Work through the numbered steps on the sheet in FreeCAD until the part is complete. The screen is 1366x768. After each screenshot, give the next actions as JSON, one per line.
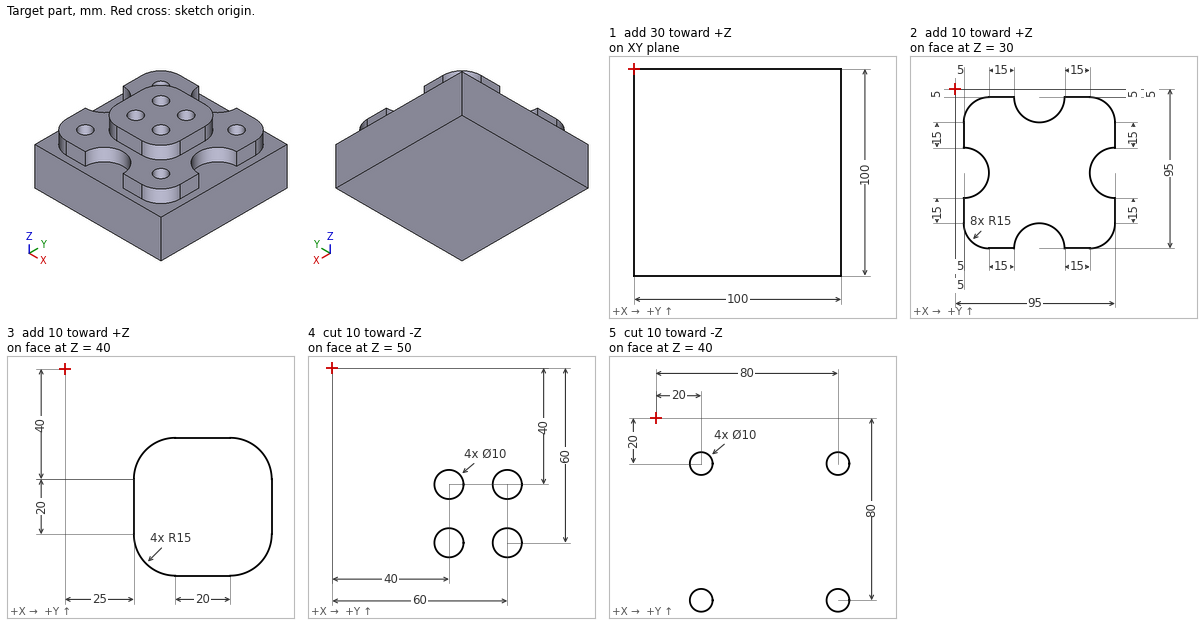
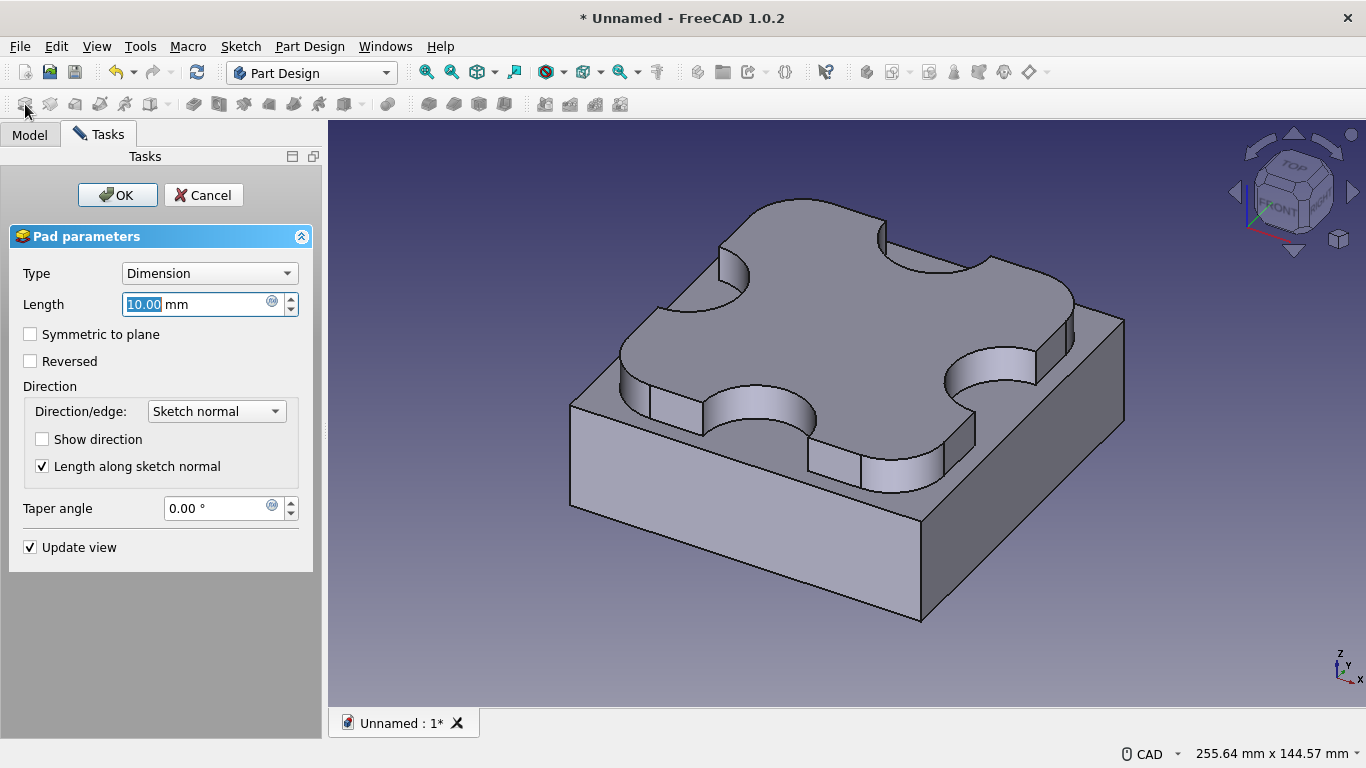
{"action": "type", "text": "10"}
{"action": "key", "text": "Tab"}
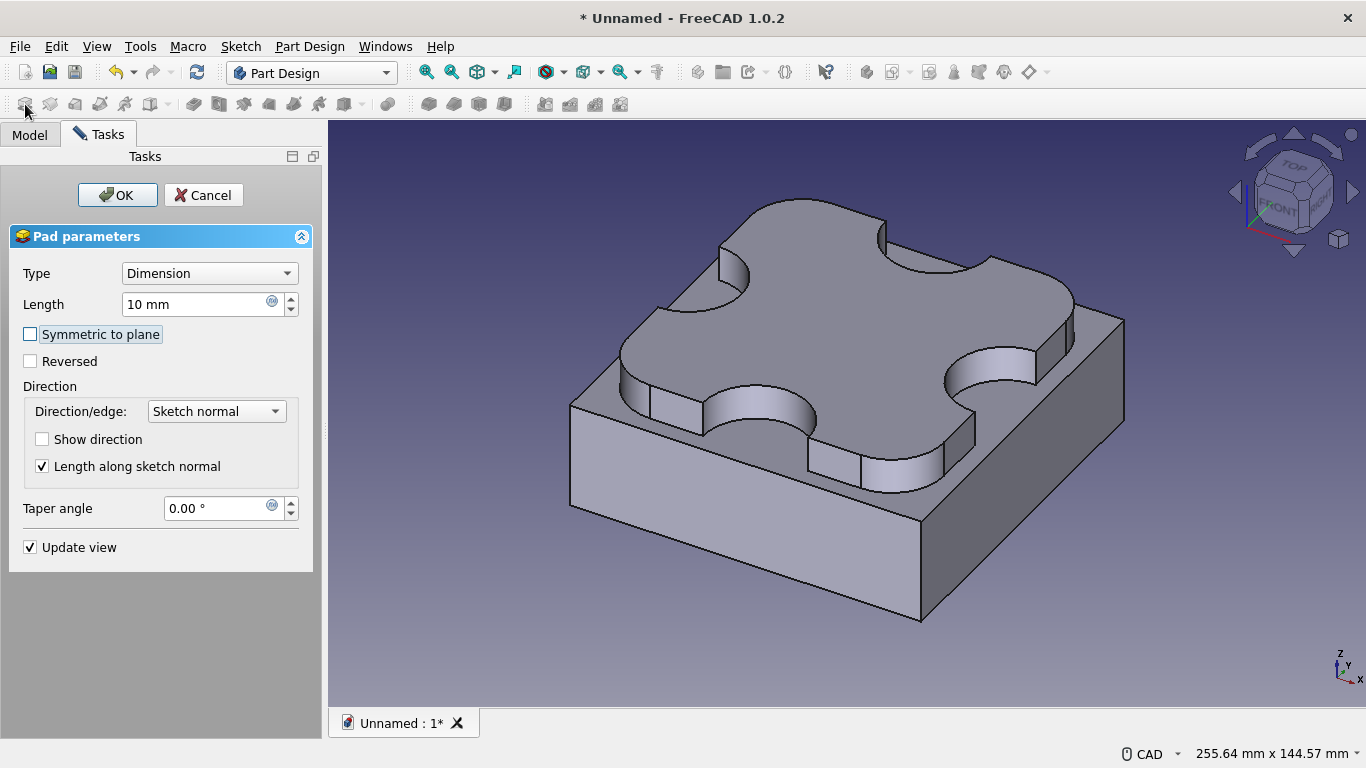
{"action": "left_click", "coordinate": [118, 195]}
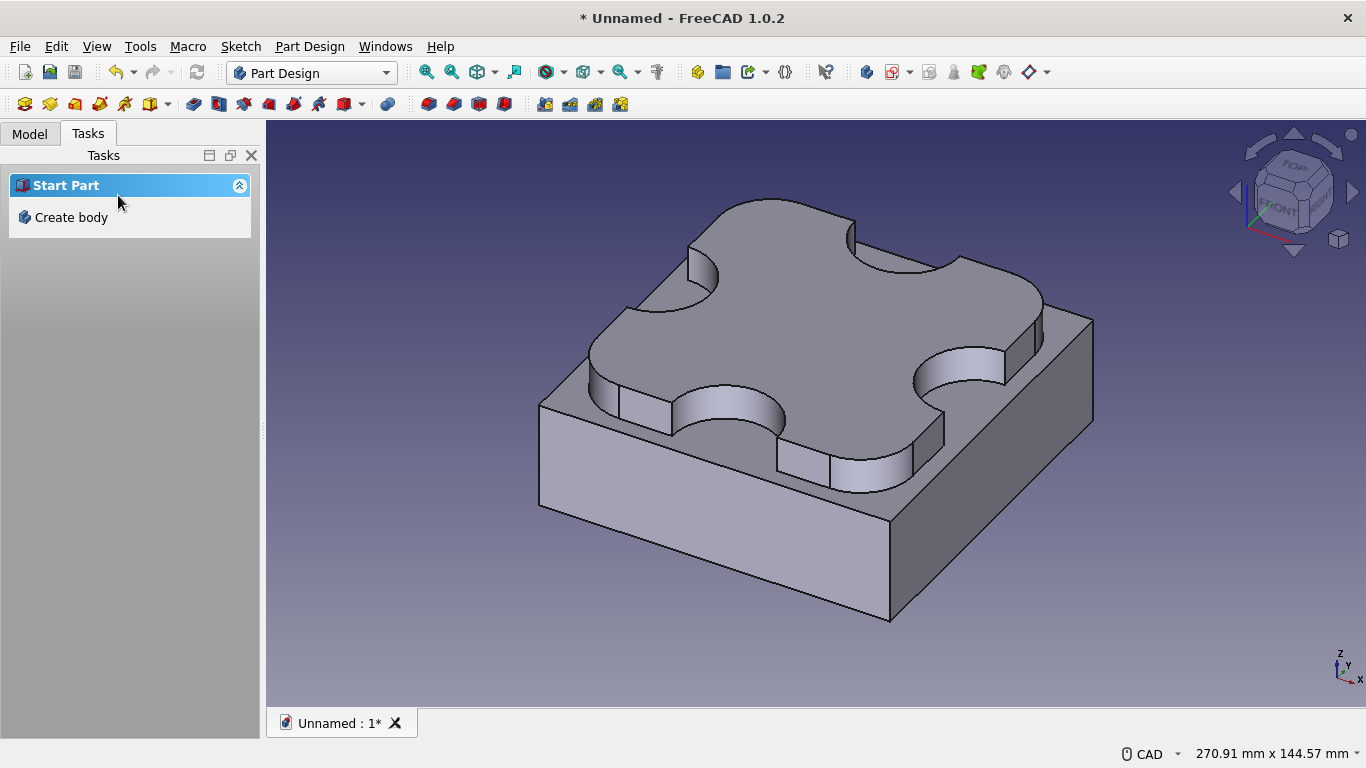
{"action": "left_click", "coordinate": [816, 328]}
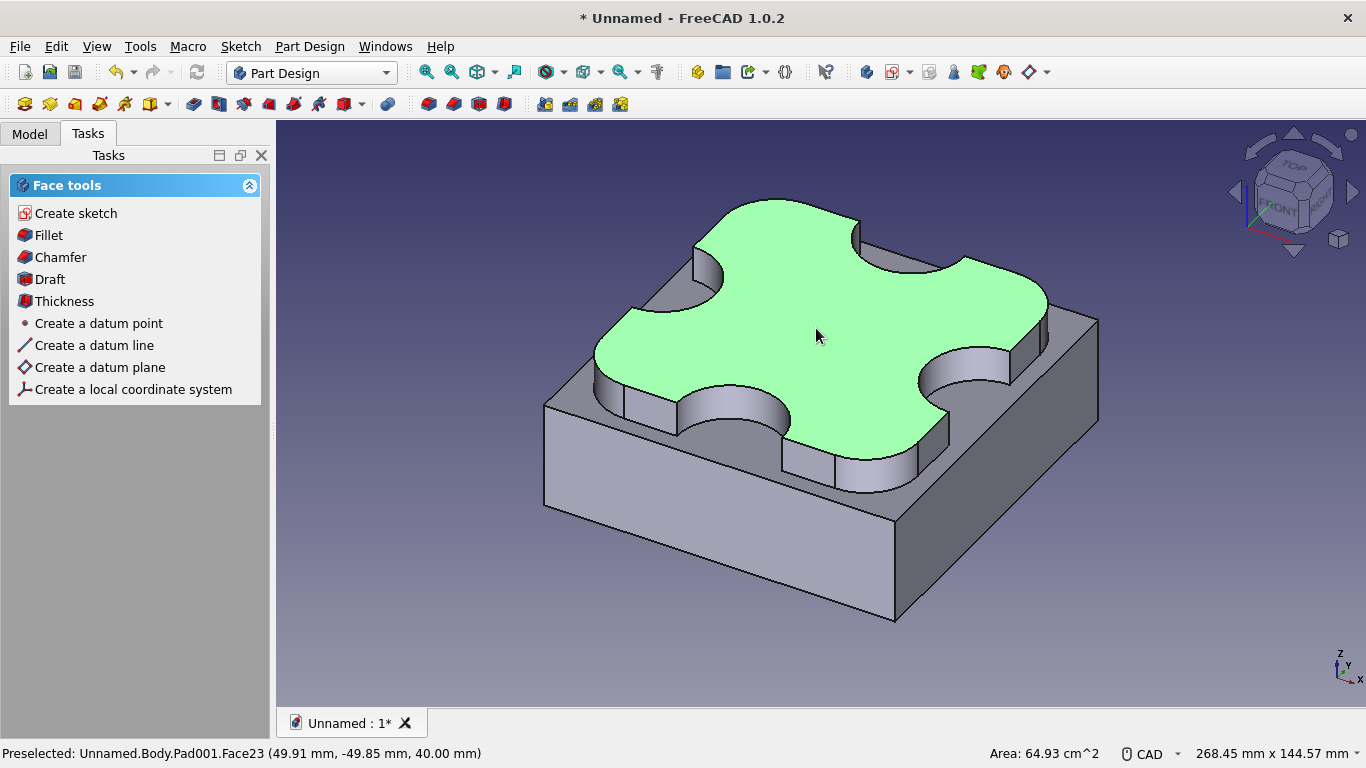
{"action": "left_click", "coordinate": [892, 72]}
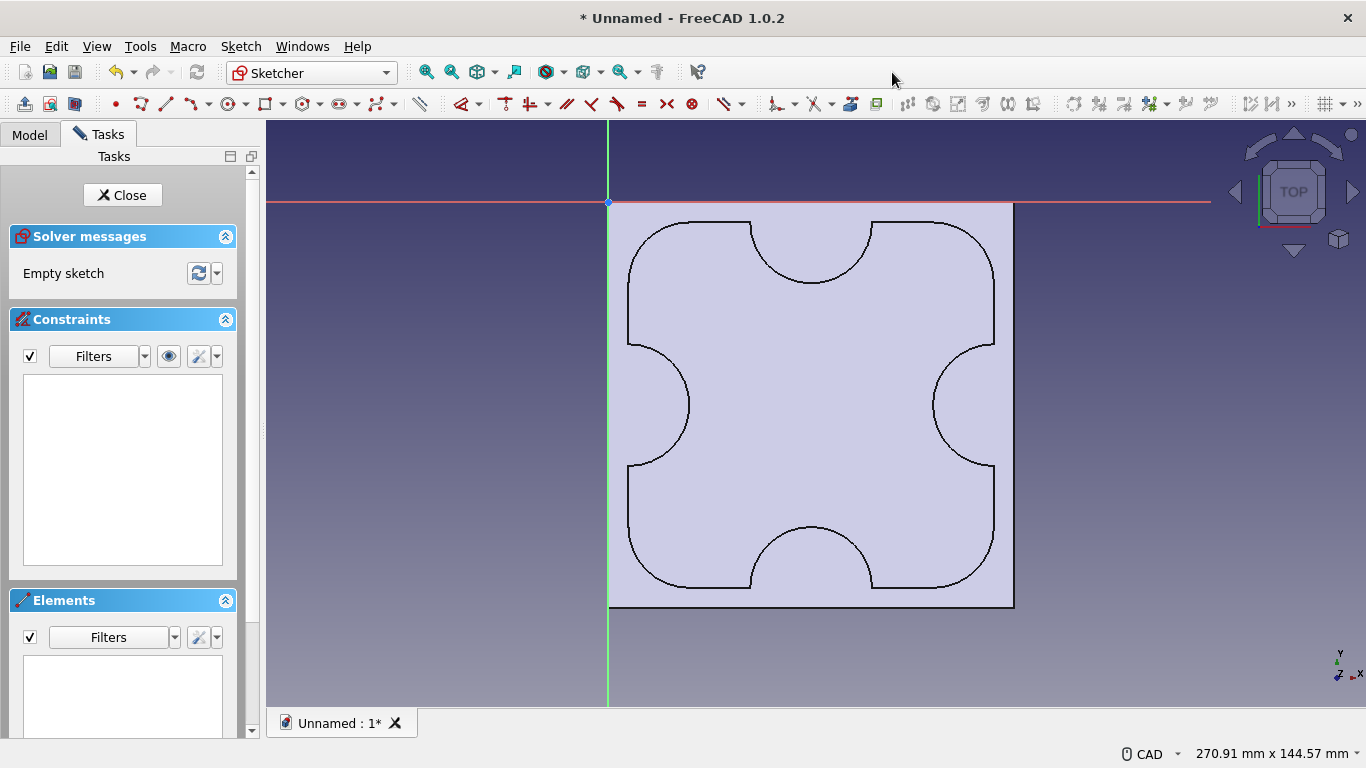
{"action": "left_click", "coordinate": [166, 104]}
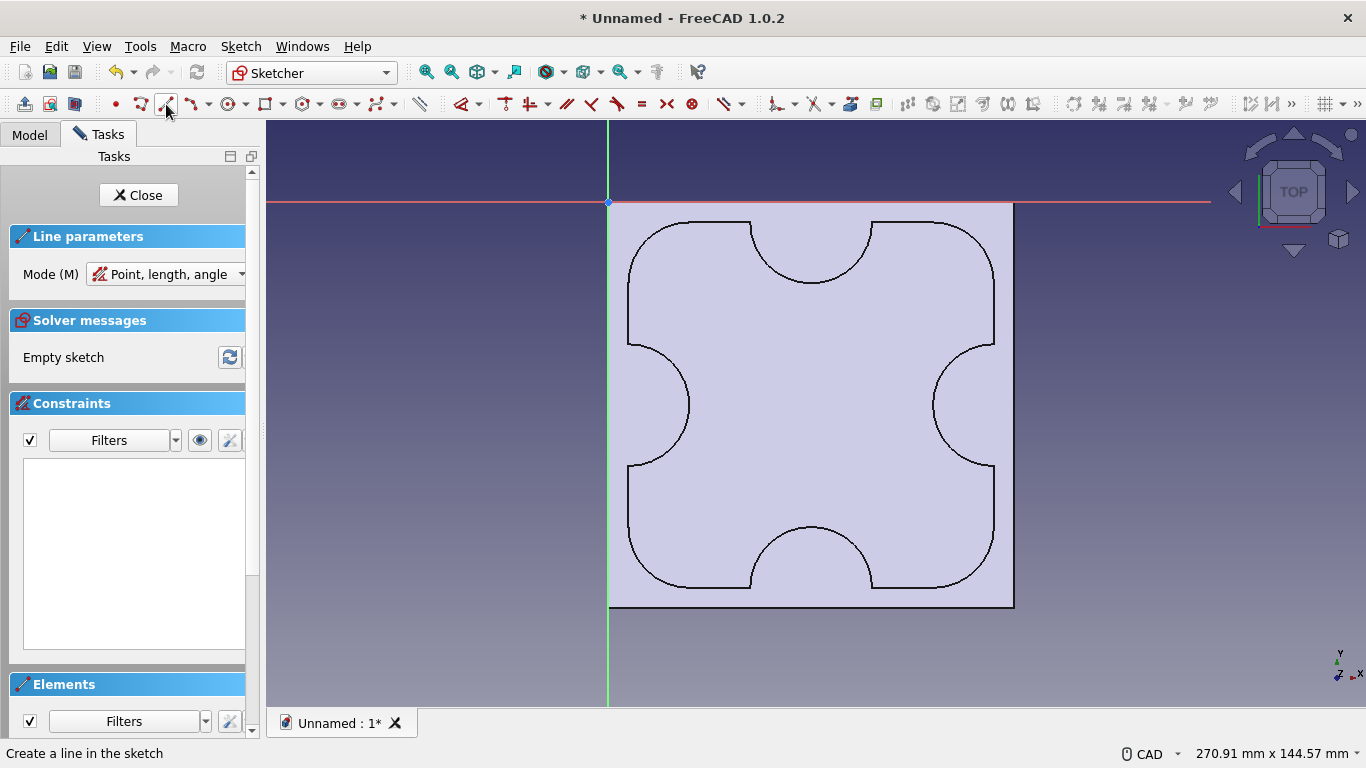
{"action": "left_click", "coordinate": [710, 365]}
{"action": "left_click", "coordinate": [710, 446]}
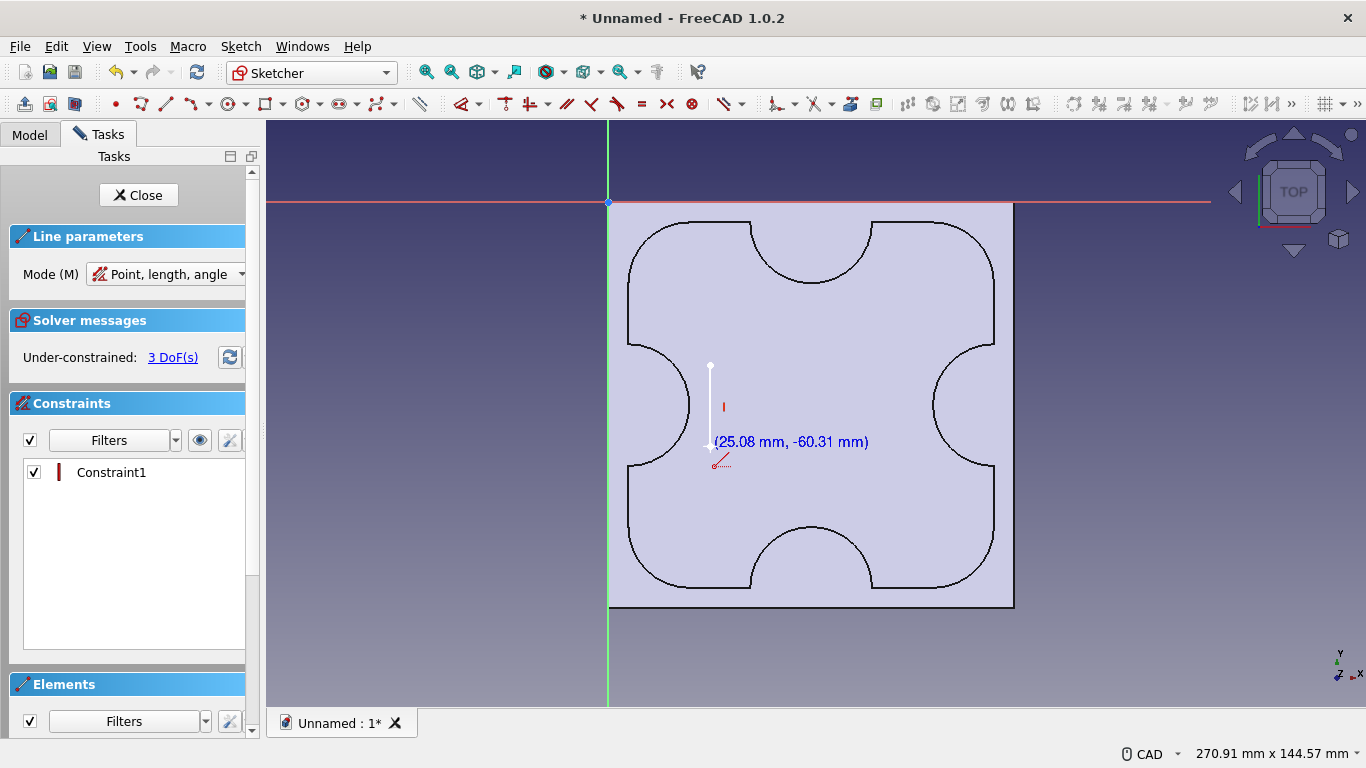
{"action": "left_click", "coordinate": [771, 507]}
{"action": "left_click", "coordinate": [852, 507]}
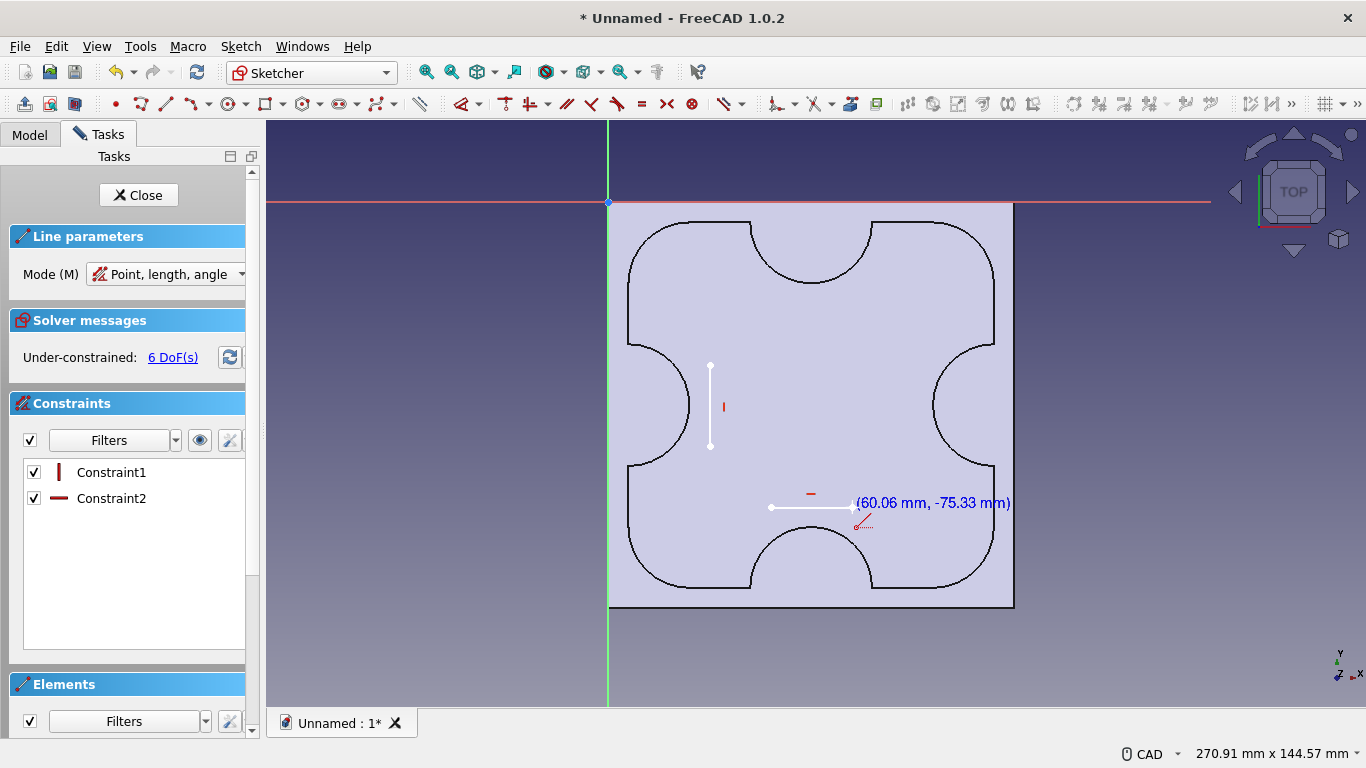
{"action": "left_click", "coordinate": [913, 446]}
{"action": "left_click", "coordinate": [913, 365]}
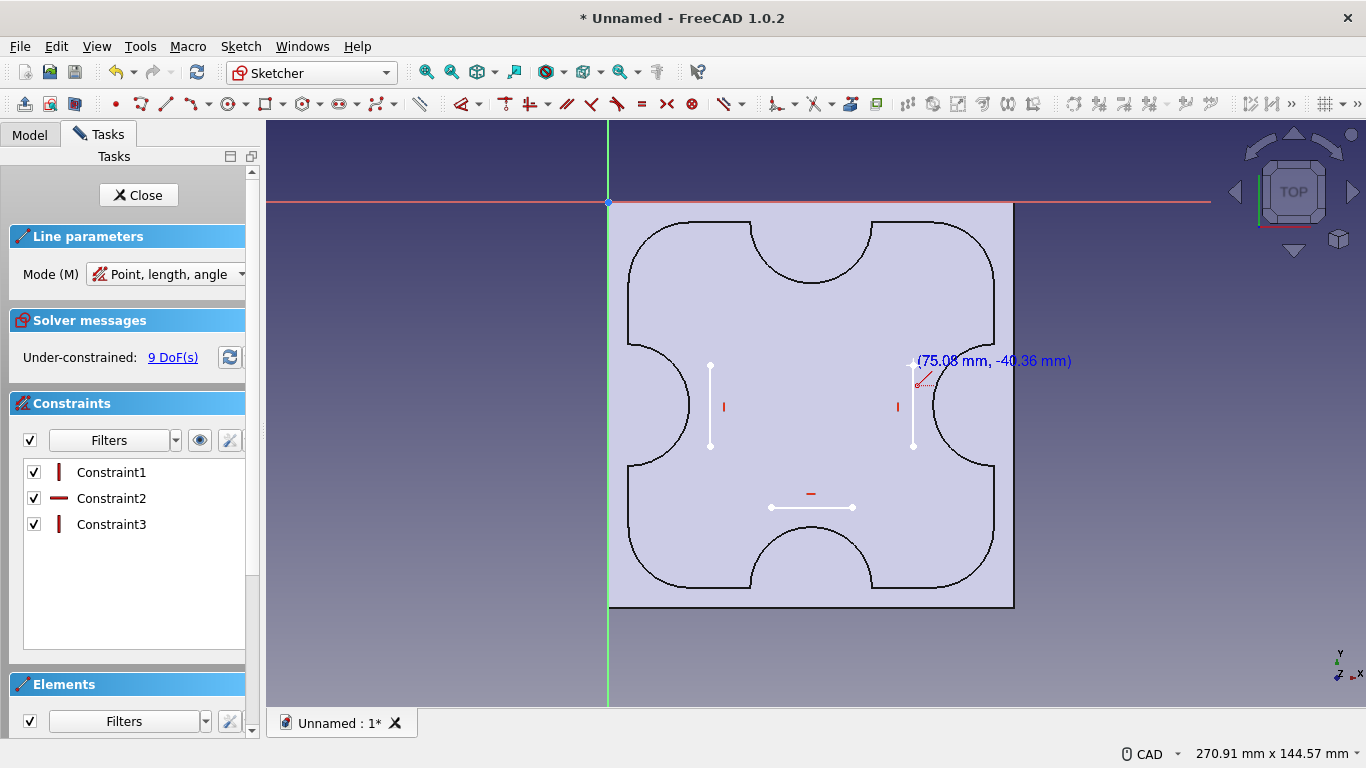
{"action": "left_click", "coordinate": [852, 304]}
{"action": "left_click", "coordinate": [771, 304]}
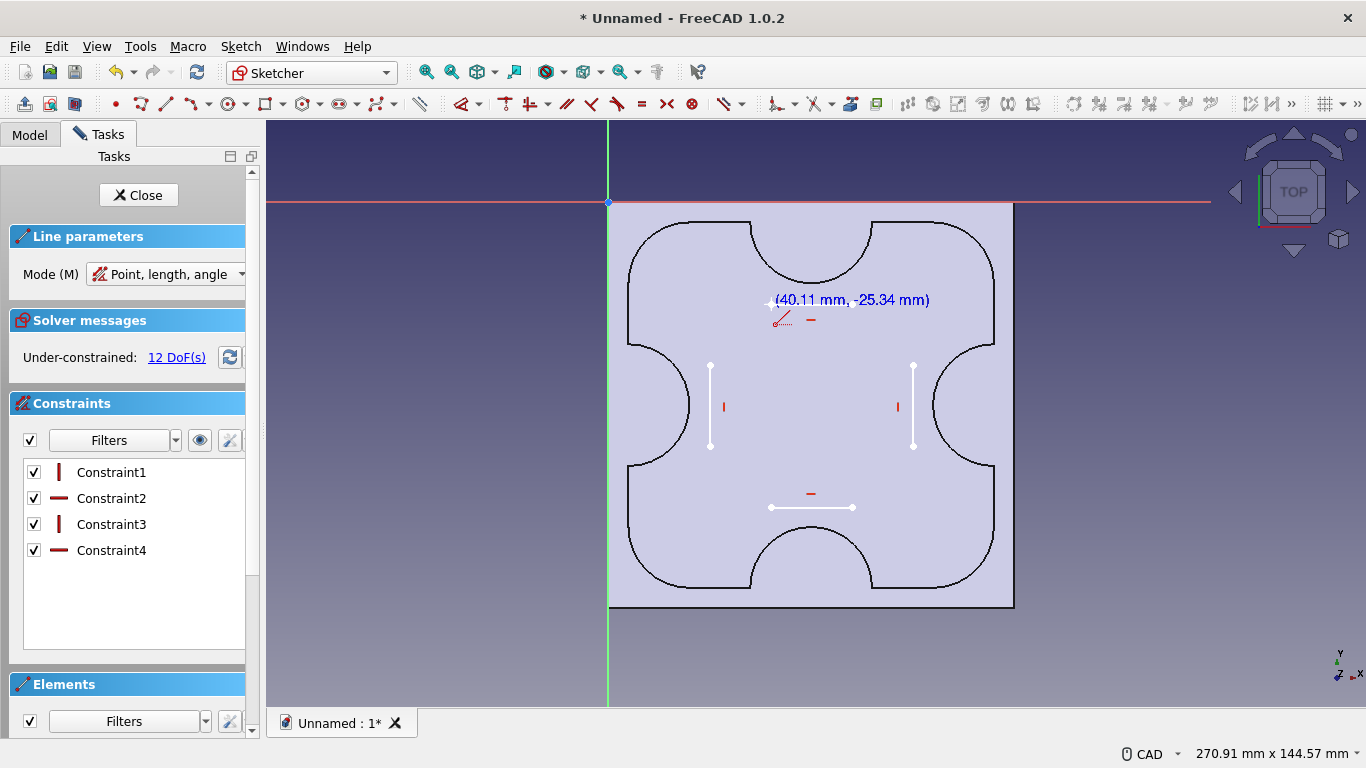
{"action": "left_click", "coordinate": [190, 104]}